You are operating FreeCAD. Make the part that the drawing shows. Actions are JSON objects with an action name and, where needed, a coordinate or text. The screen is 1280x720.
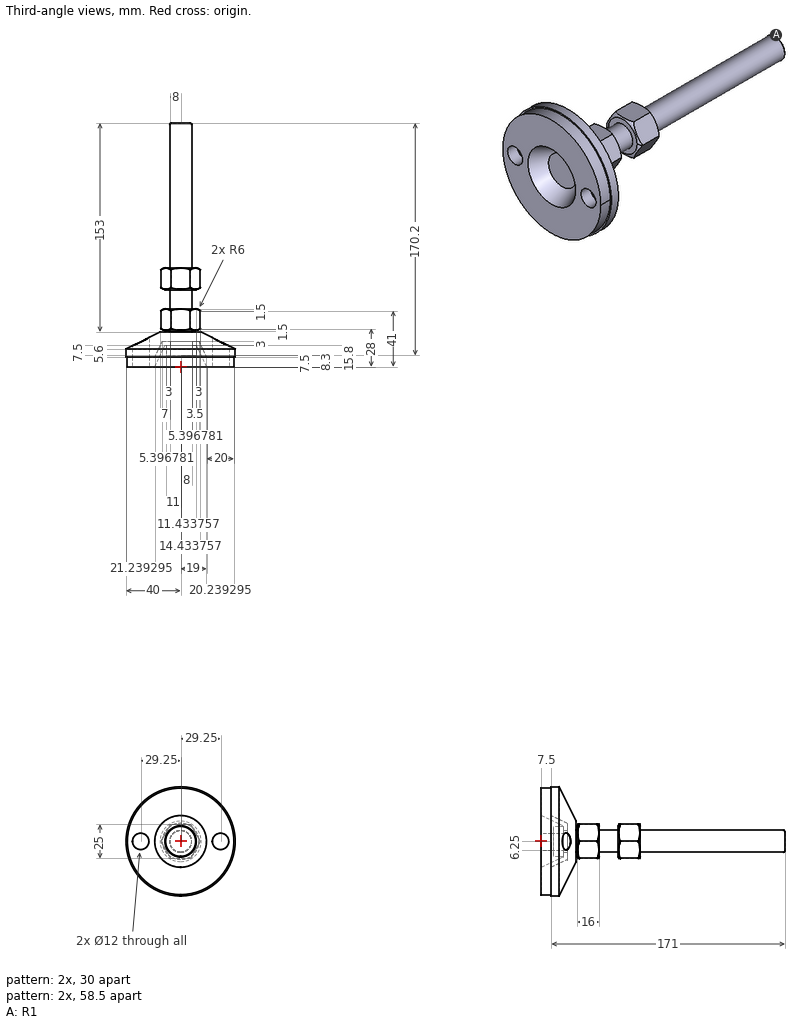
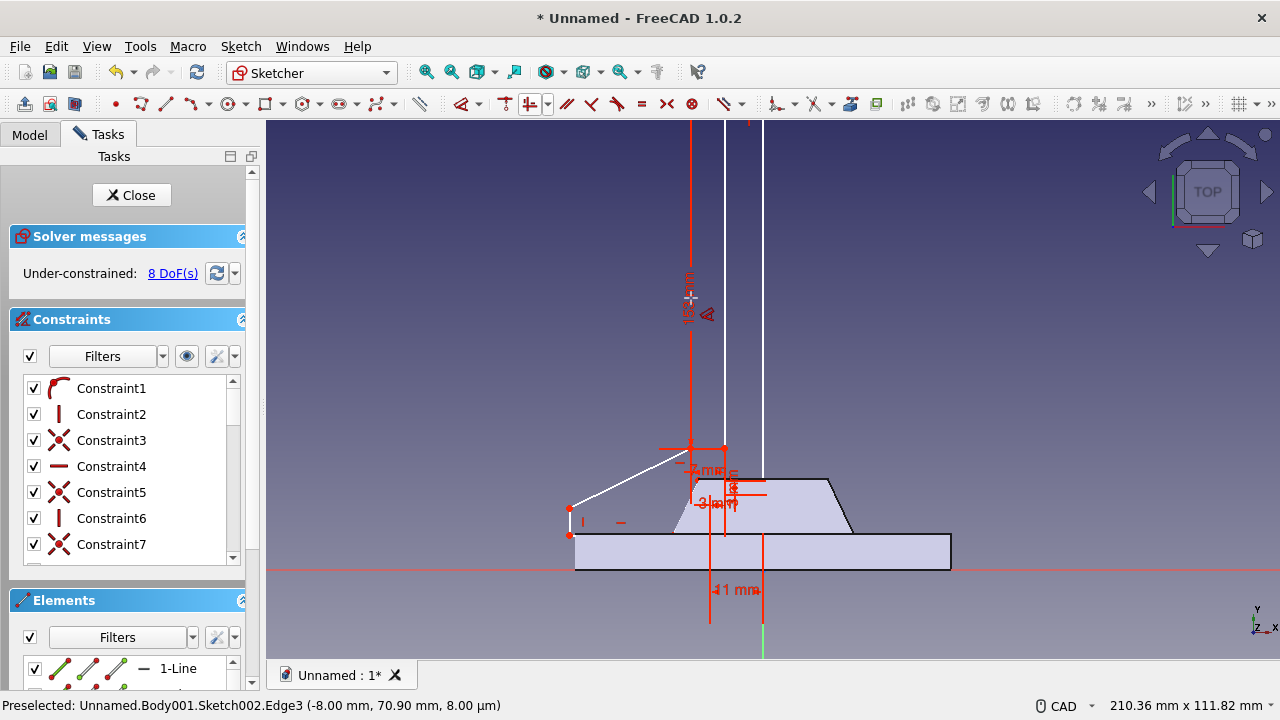
{"action": "scroll", "coordinate": [570, 519], "scroll_direction": "up", "scroll_amount": 2}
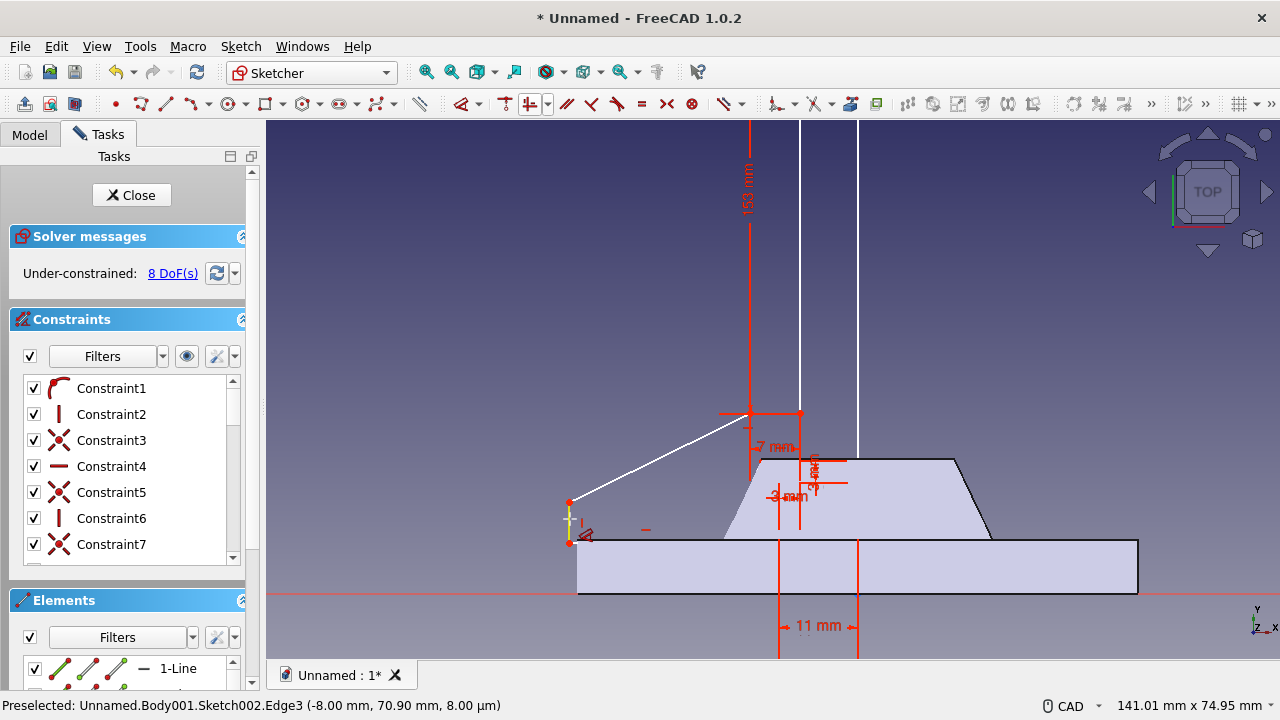
{"action": "left_click", "coordinate": [569, 519]}
{"action": "left_click", "coordinate": [535, 523]}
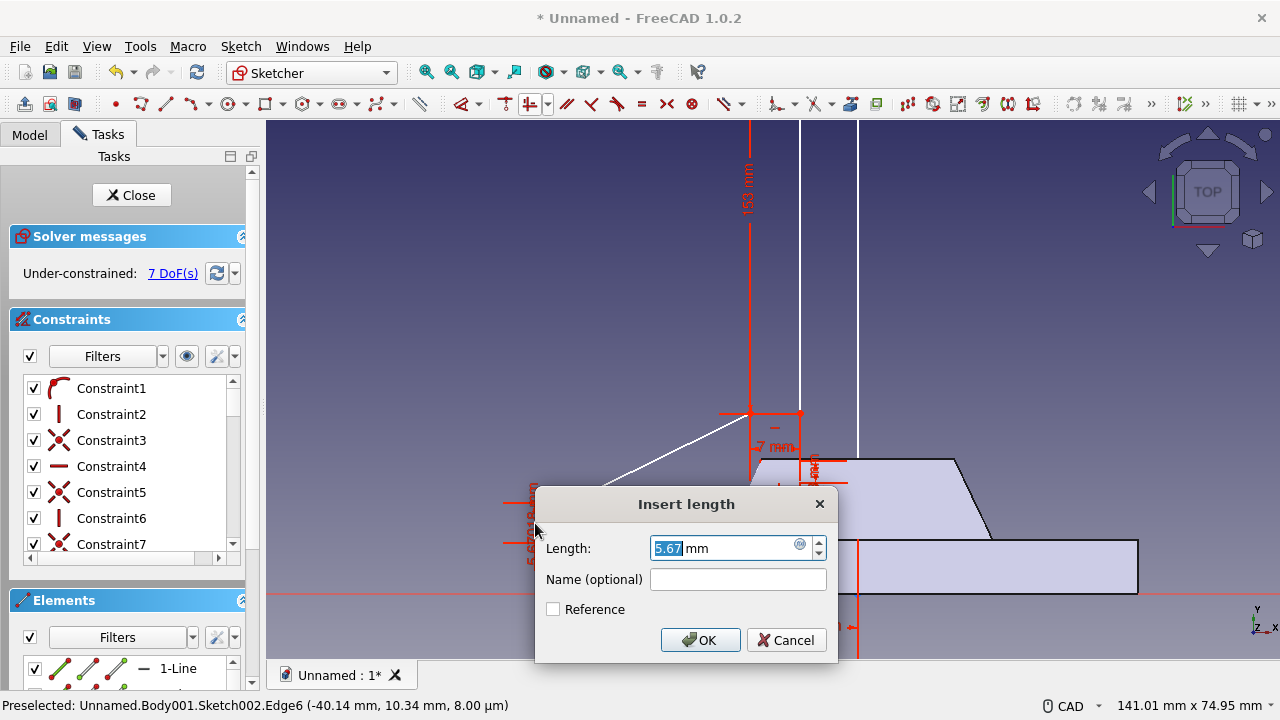
{"action": "type", "text": "5.6"}
{"action": "key", "text": "Return"}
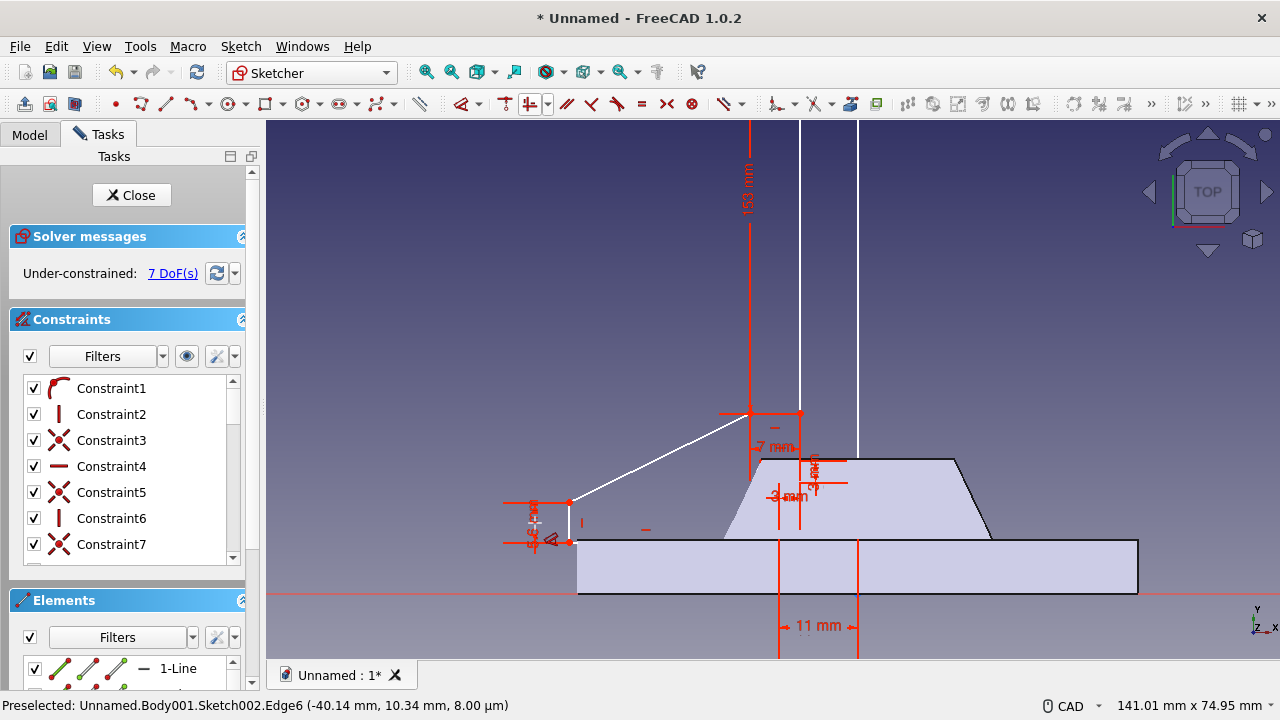
{"action": "left_click", "coordinate": [779, 500]}
{"action": "left_click", "coordinate": [813, 524]}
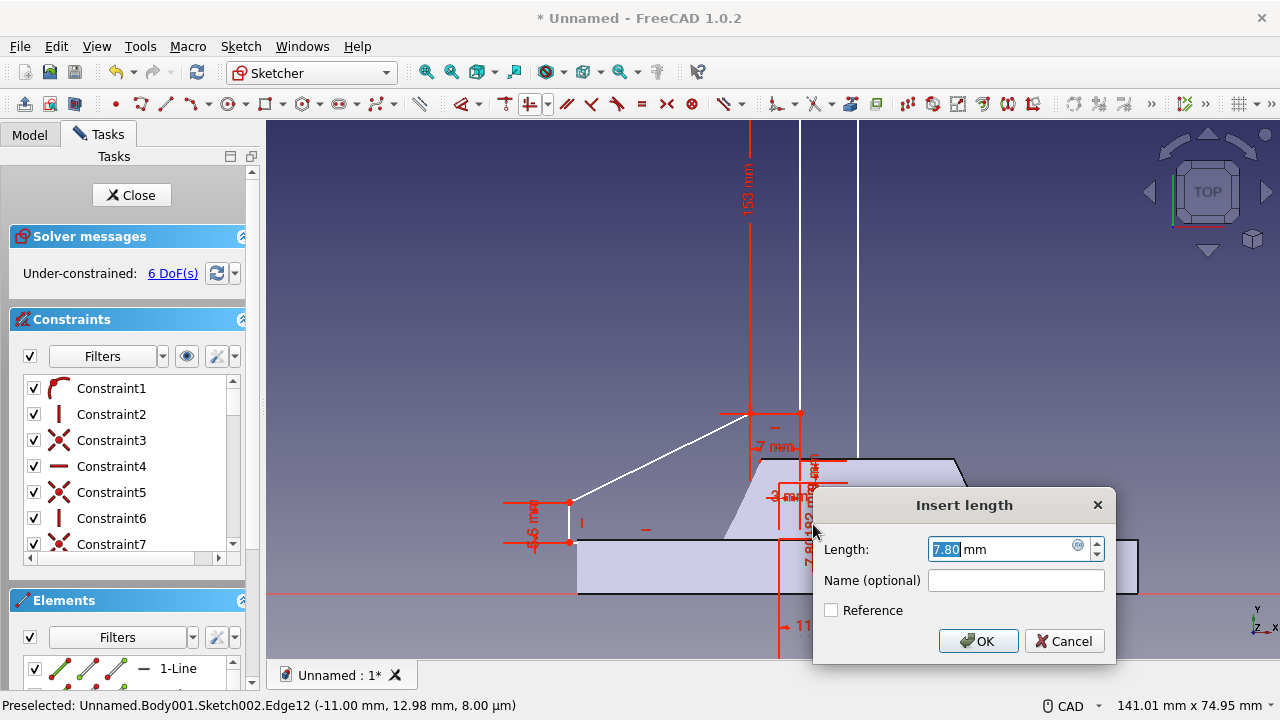
{"action": "type", "text": "7.5"}
{"action": "key", "text": "Return"}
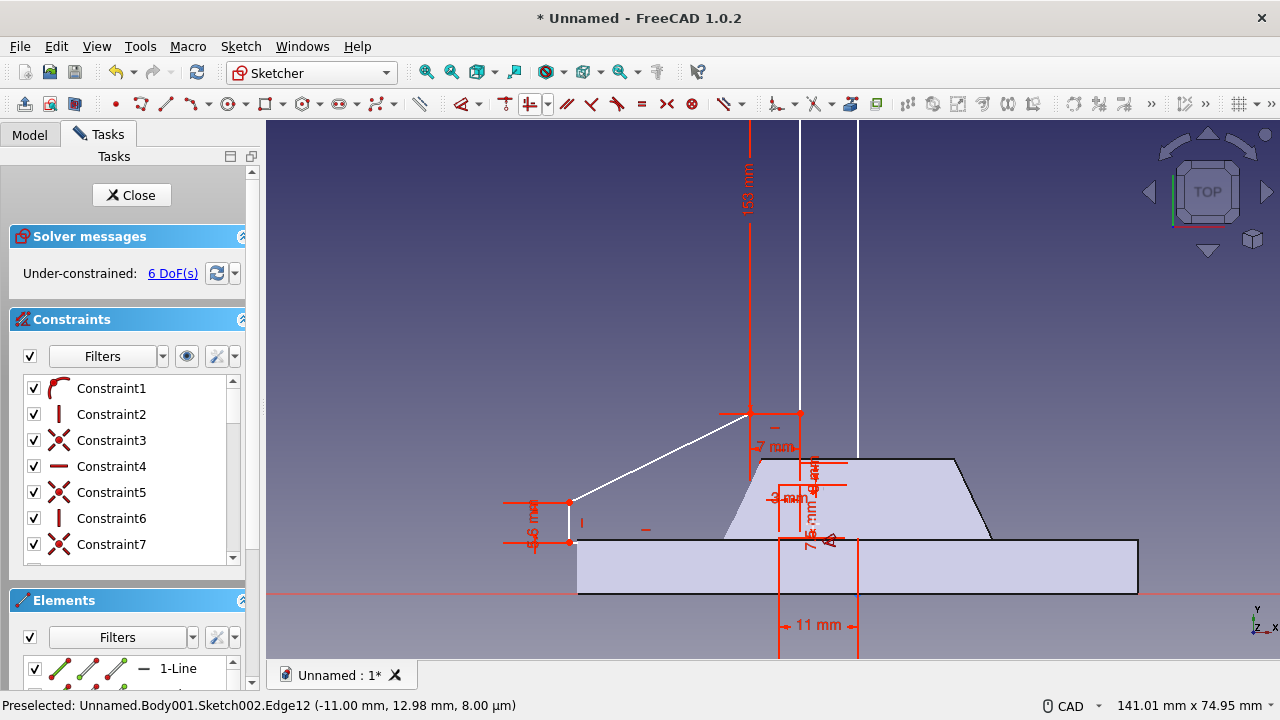
{"action": "scroll", "coordinate": [701, 533], "scroll_direction": "down", "scroll_amount": 7}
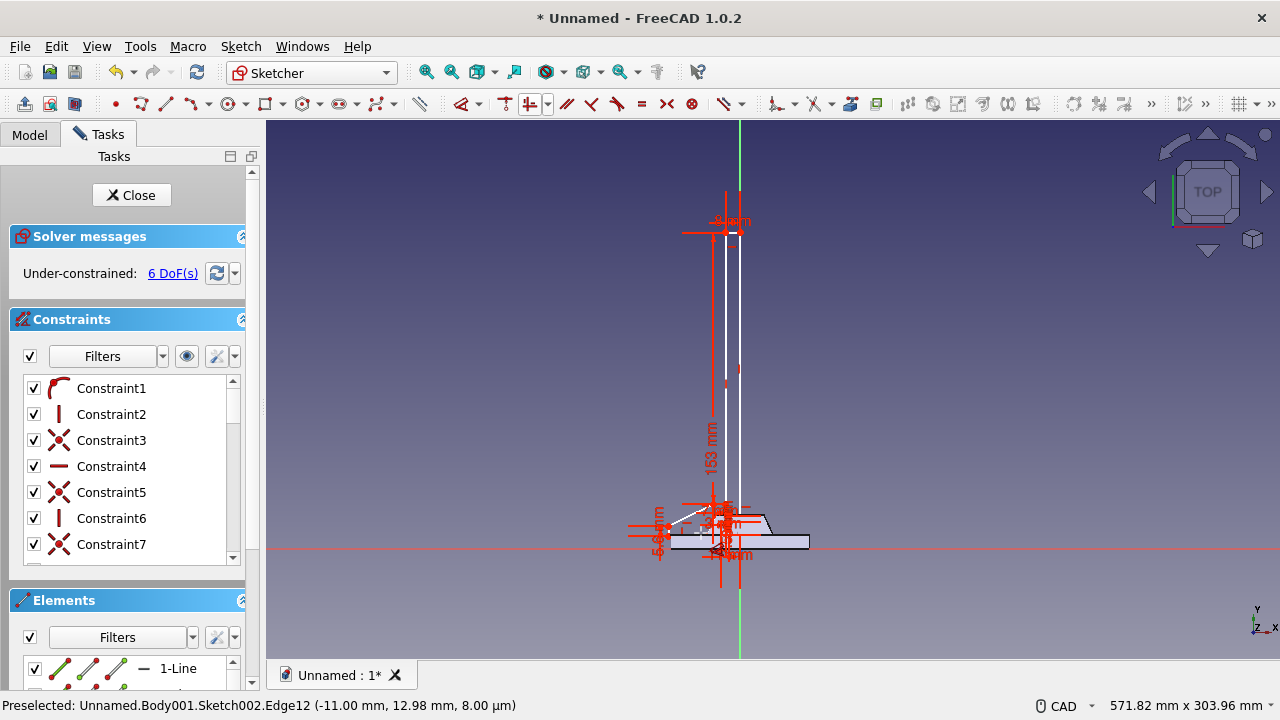
{"action": "scroll", "coordinate": [669, 526], "scroll_direction": "up", "scroll_amount": 2}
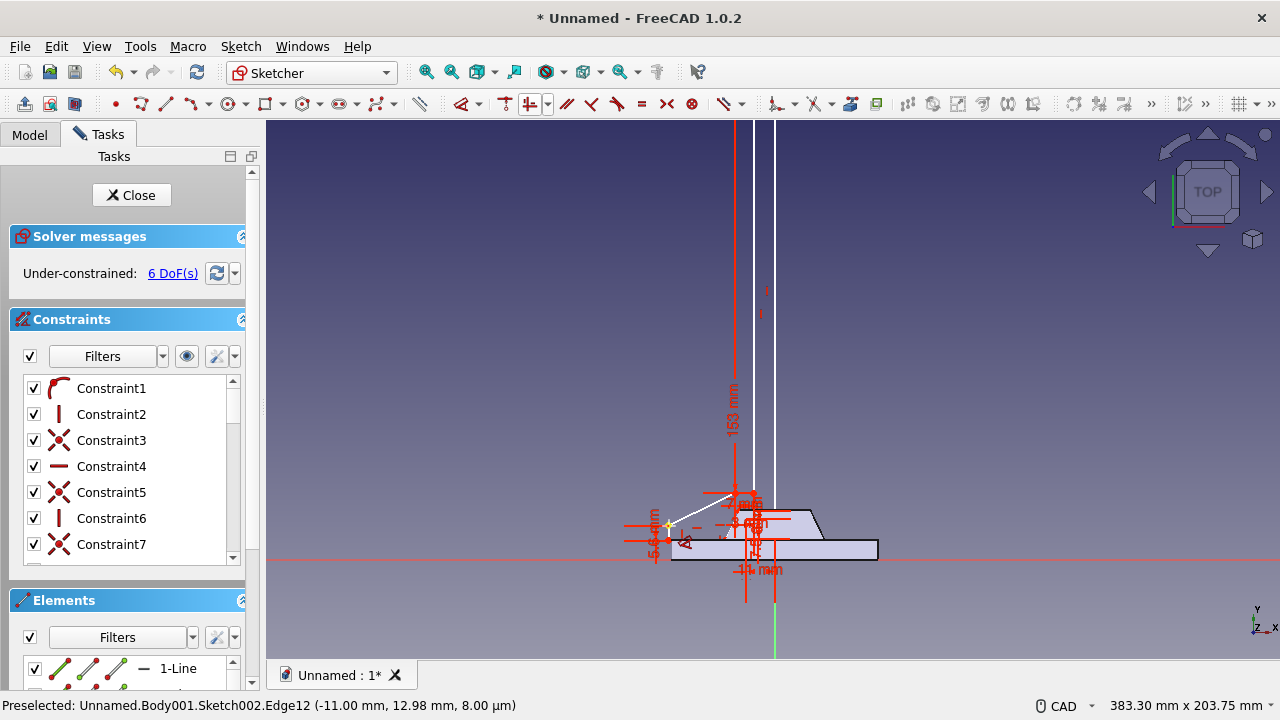
{"action": "left_click", "coordinate": [669, 526]}
{"action": "left_click", "coordinate": [722, 594]}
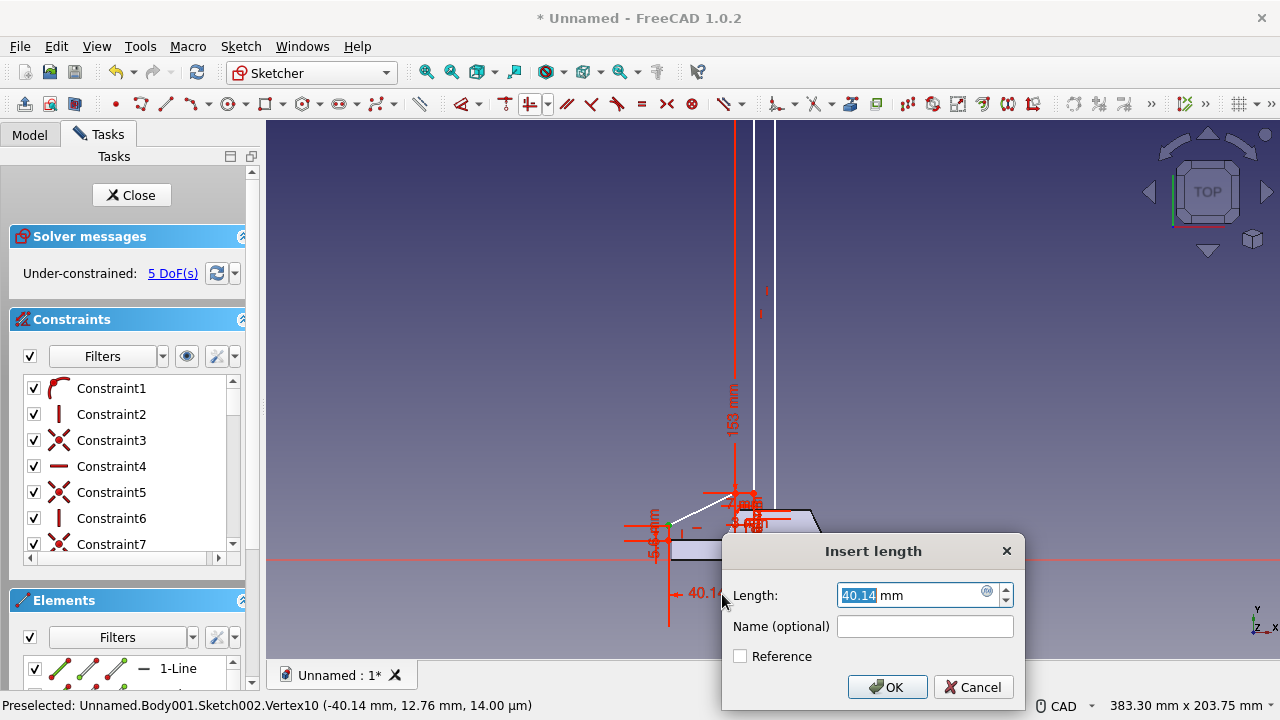
{"action": "type", "text": "40"}
{"action": "key", "text": "Return"}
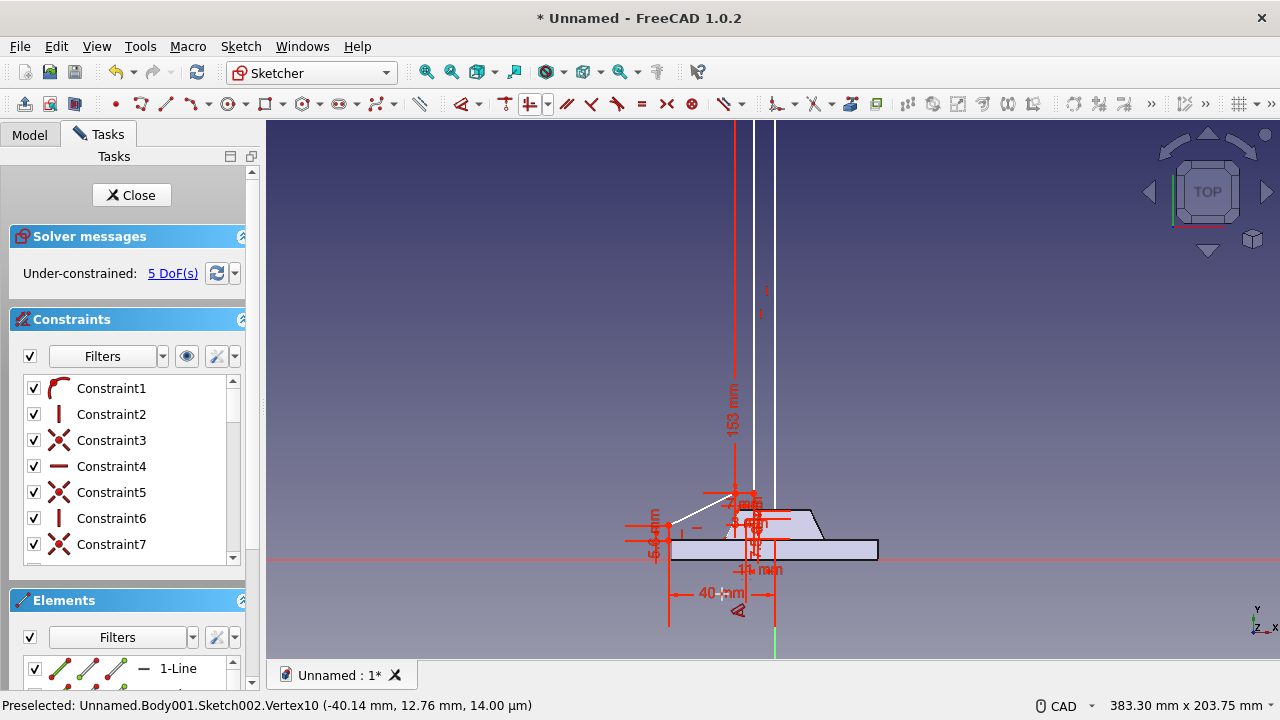
{"action": "scroll", "coordinate": [775, 539], "scroll_direction": "up", "scroll_amount": 3}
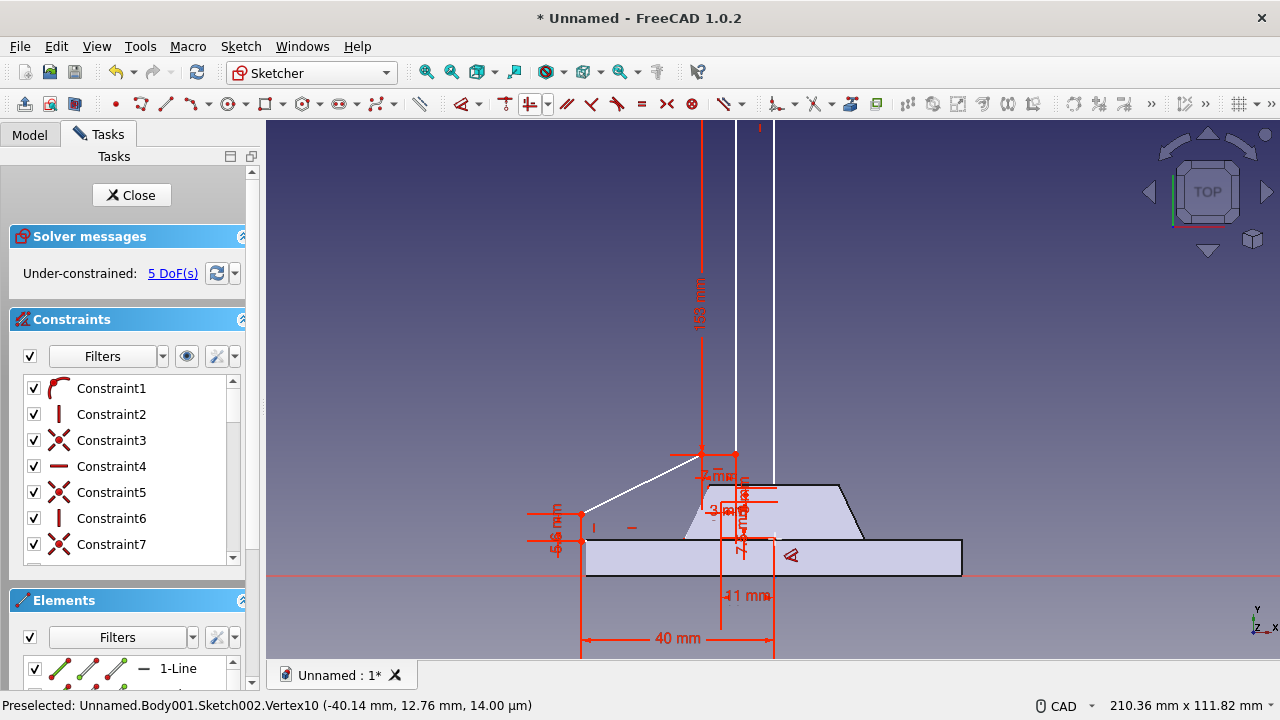
{"action": "left_click", "coordinate": [774, 538]}
{"action": "left_click", "coordinate": [808, 557]}